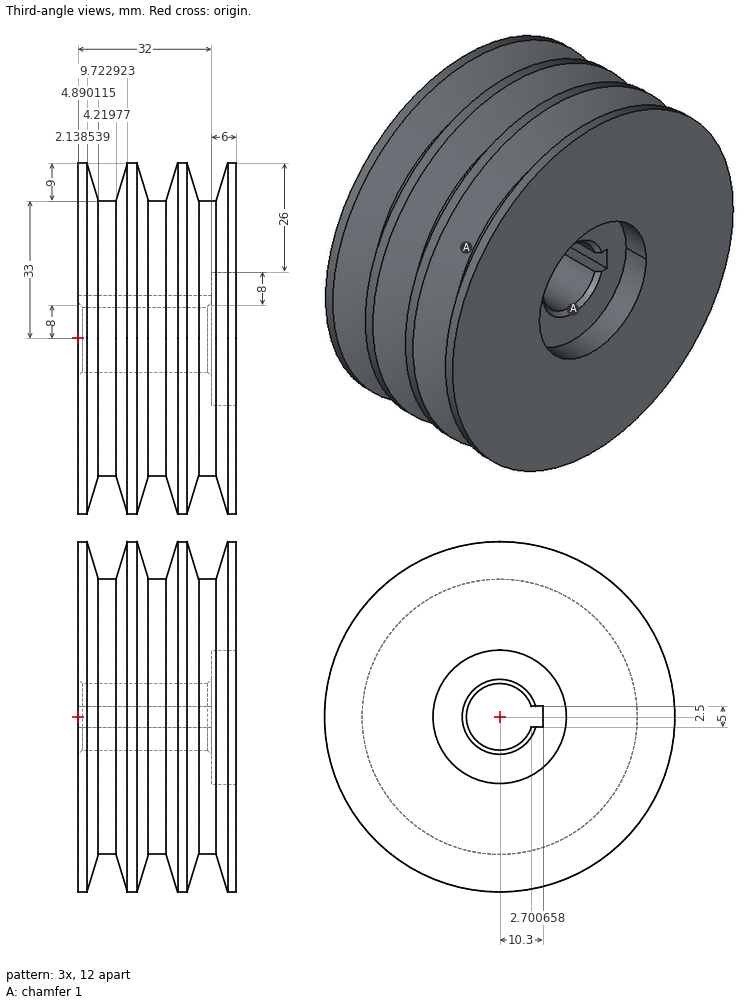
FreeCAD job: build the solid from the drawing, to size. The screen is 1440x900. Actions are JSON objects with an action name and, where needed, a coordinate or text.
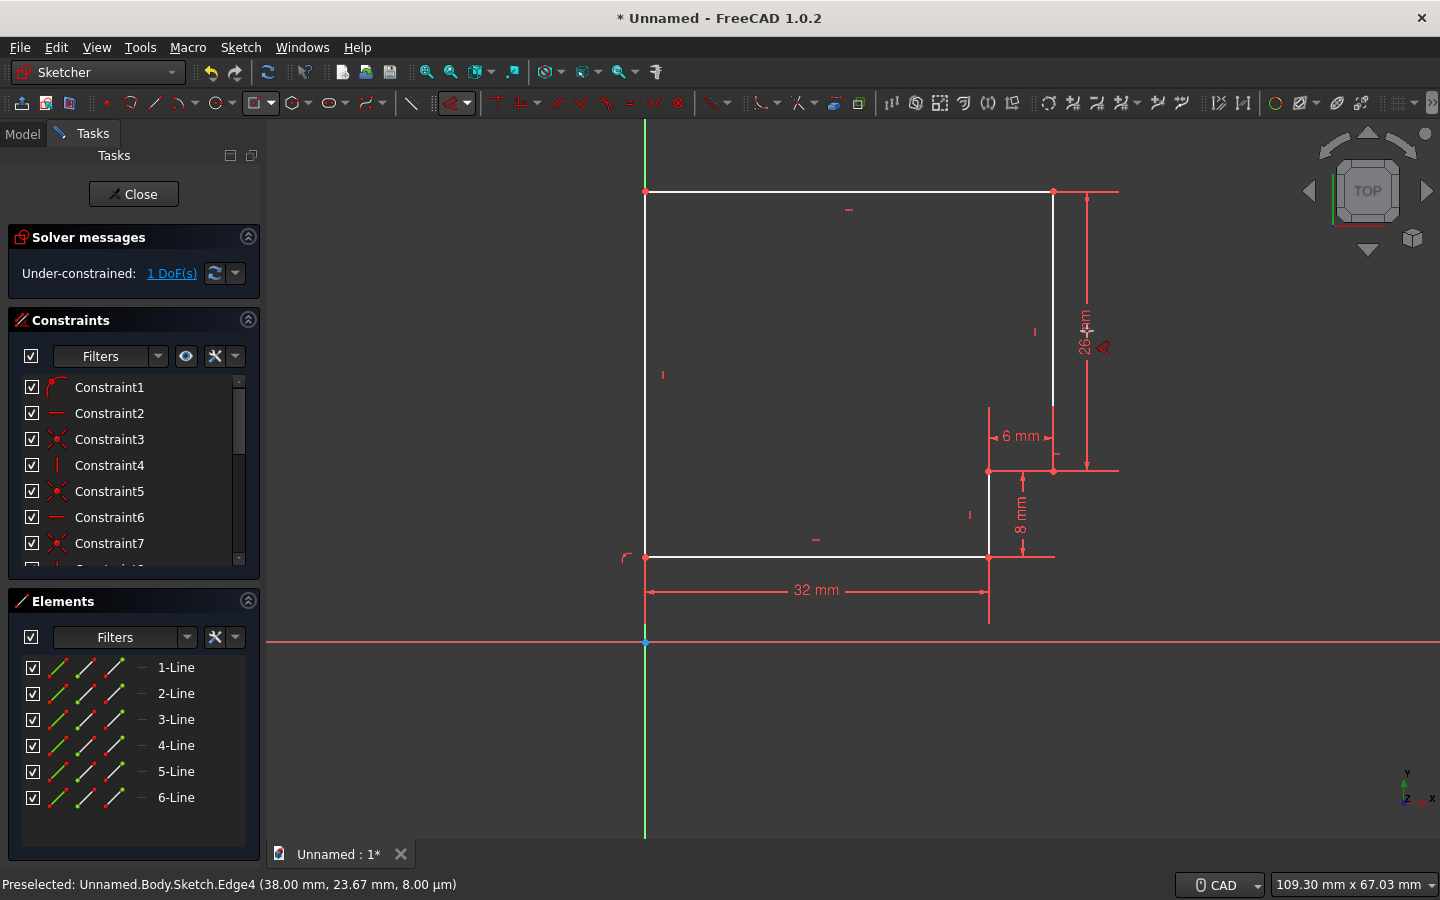
{"action": "left_click", "coordinate": [645, 557]}
{"action": "left_click", "coordinate": [611, 600]}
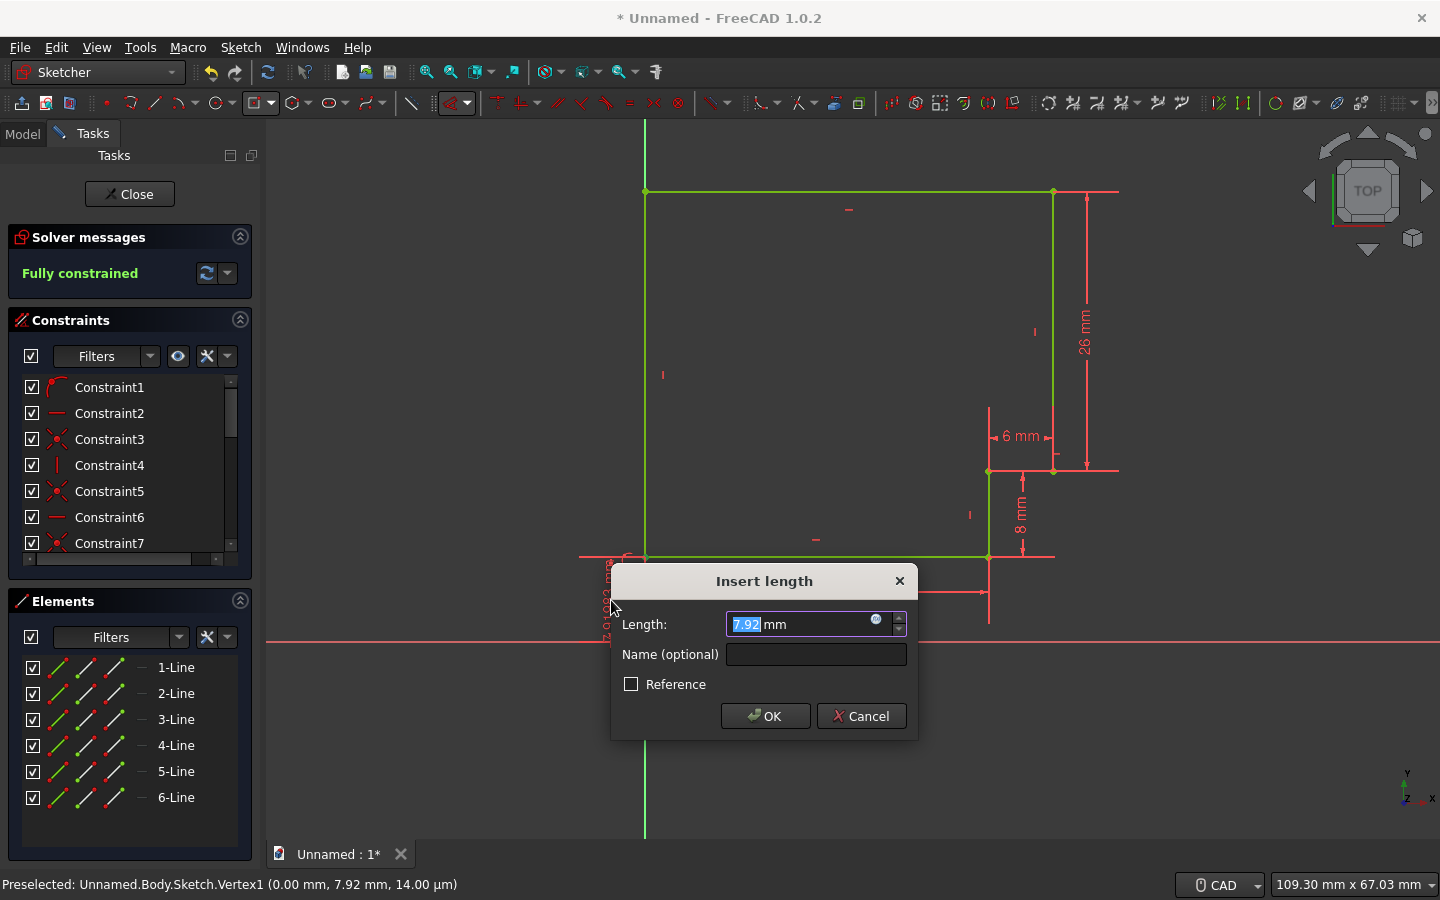
{"action": "type", "text": "8"}
{"action": "key", "text": "Return"}
{"action": "key", "text": "Escape"}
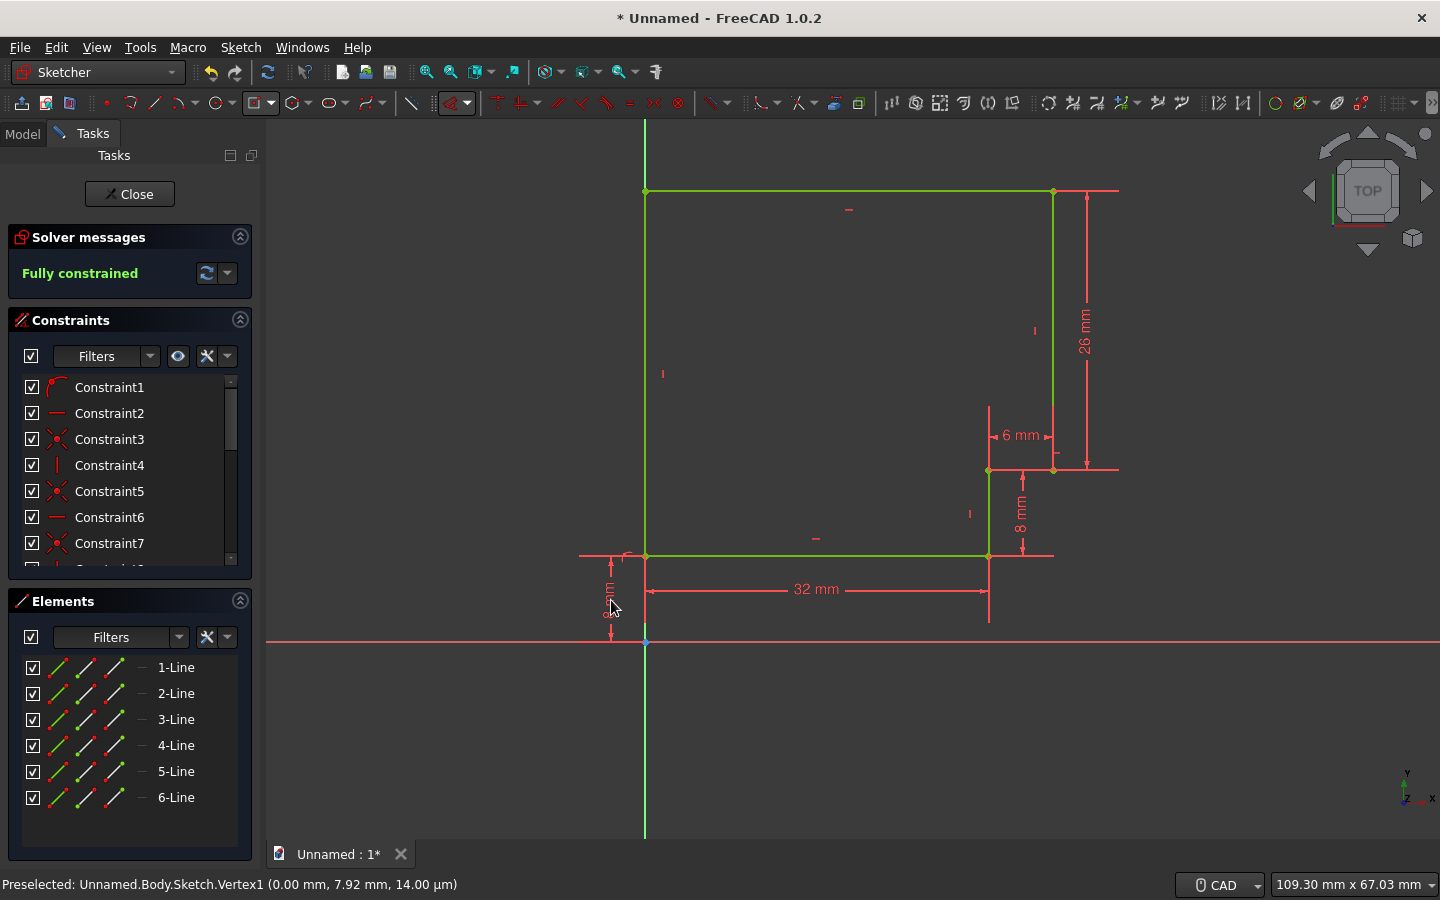
{"action": "left_click", "coordinate": [130, 194]}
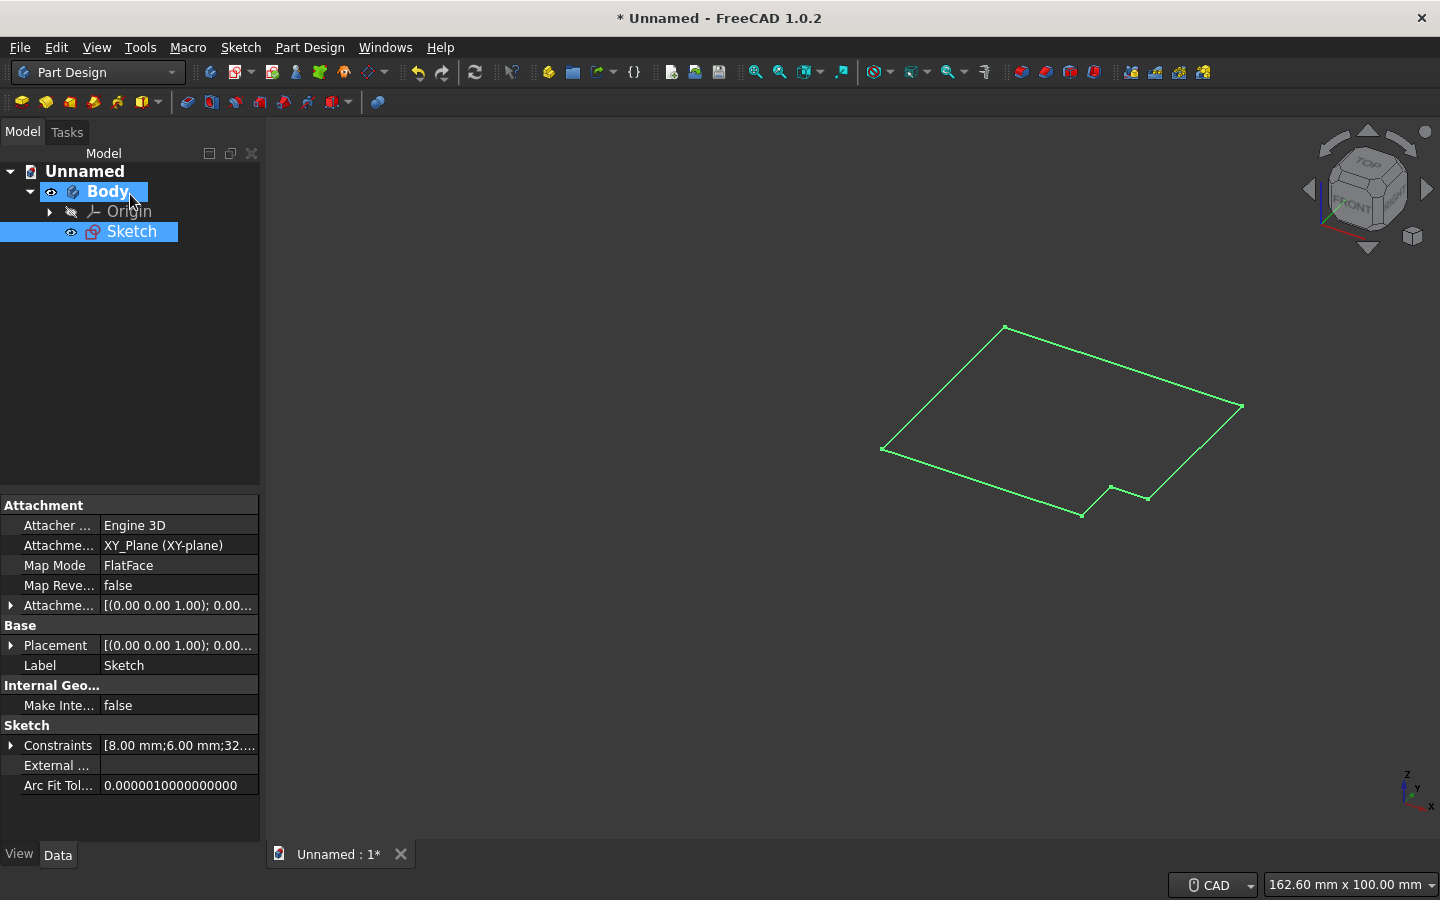
{"action": "left_click", "coordinate": [46, 102]}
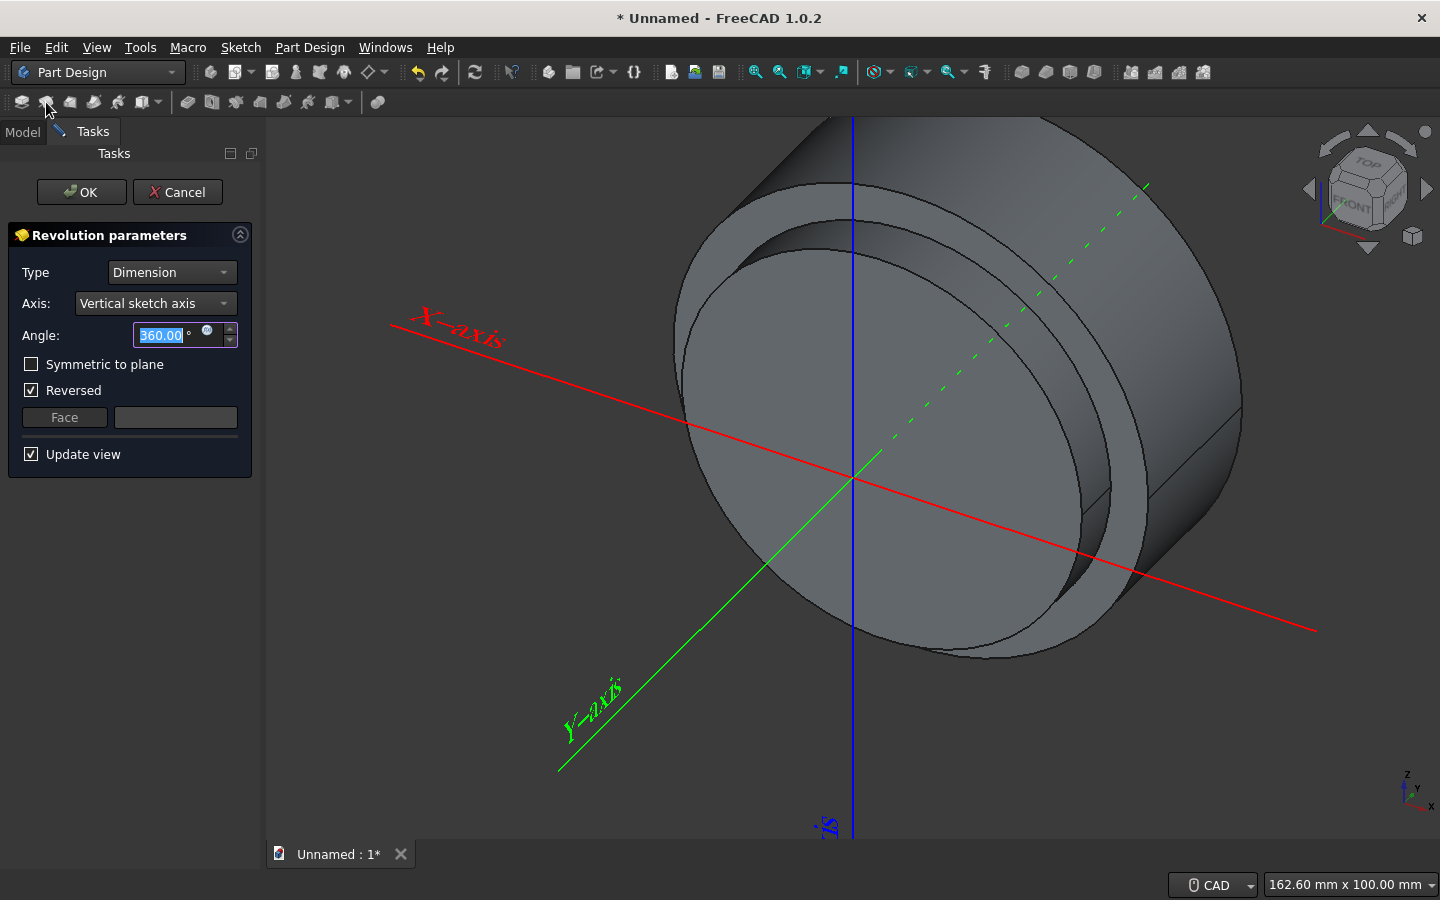
{"action": "left_click", "coordinate": [156, 304]}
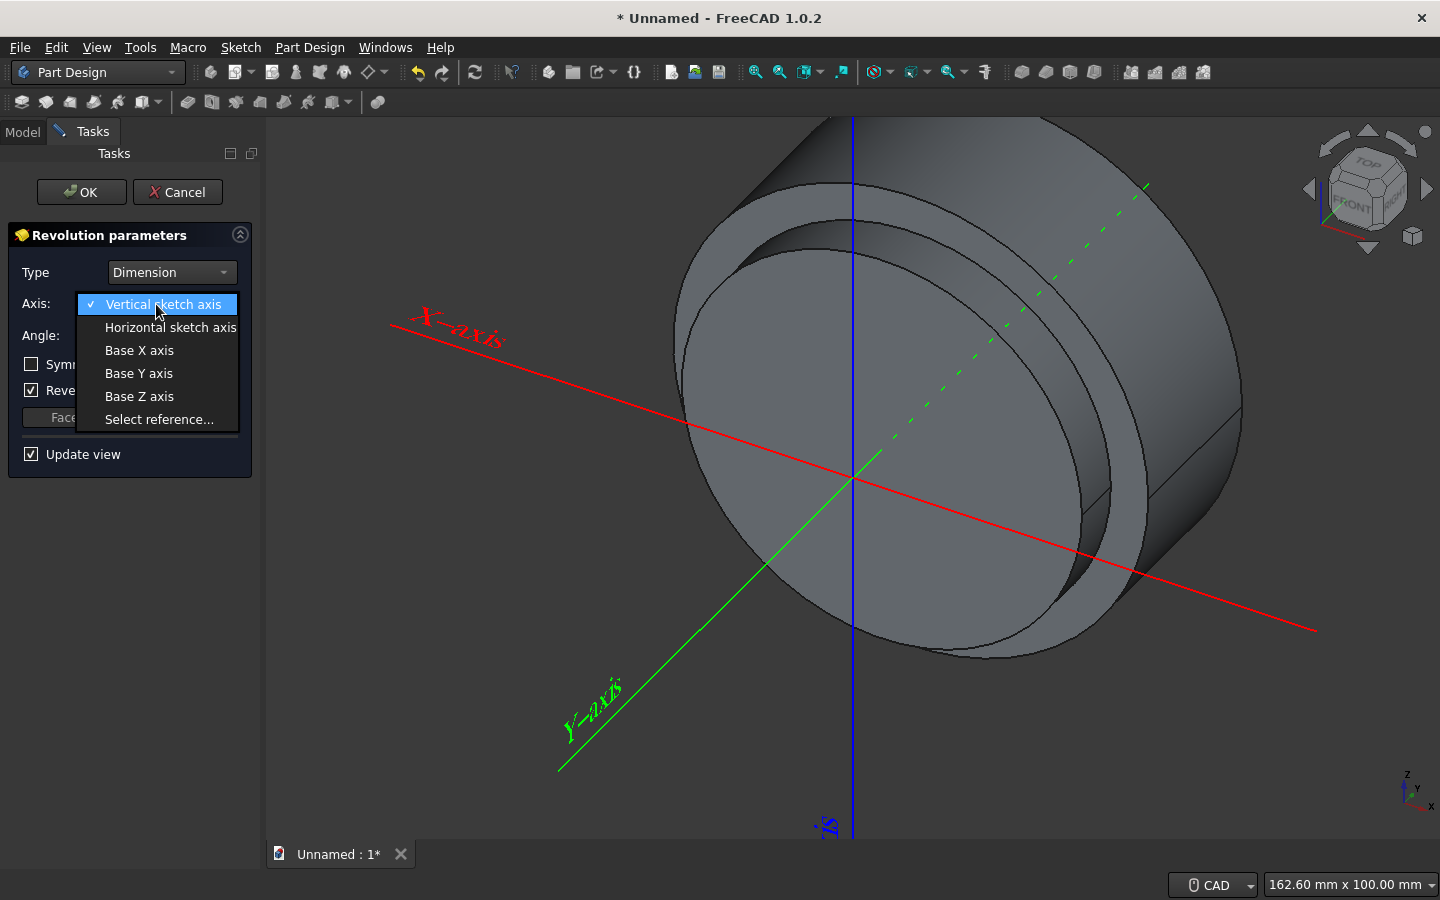
{"action": "left_click", "coordinate": [156, 328]}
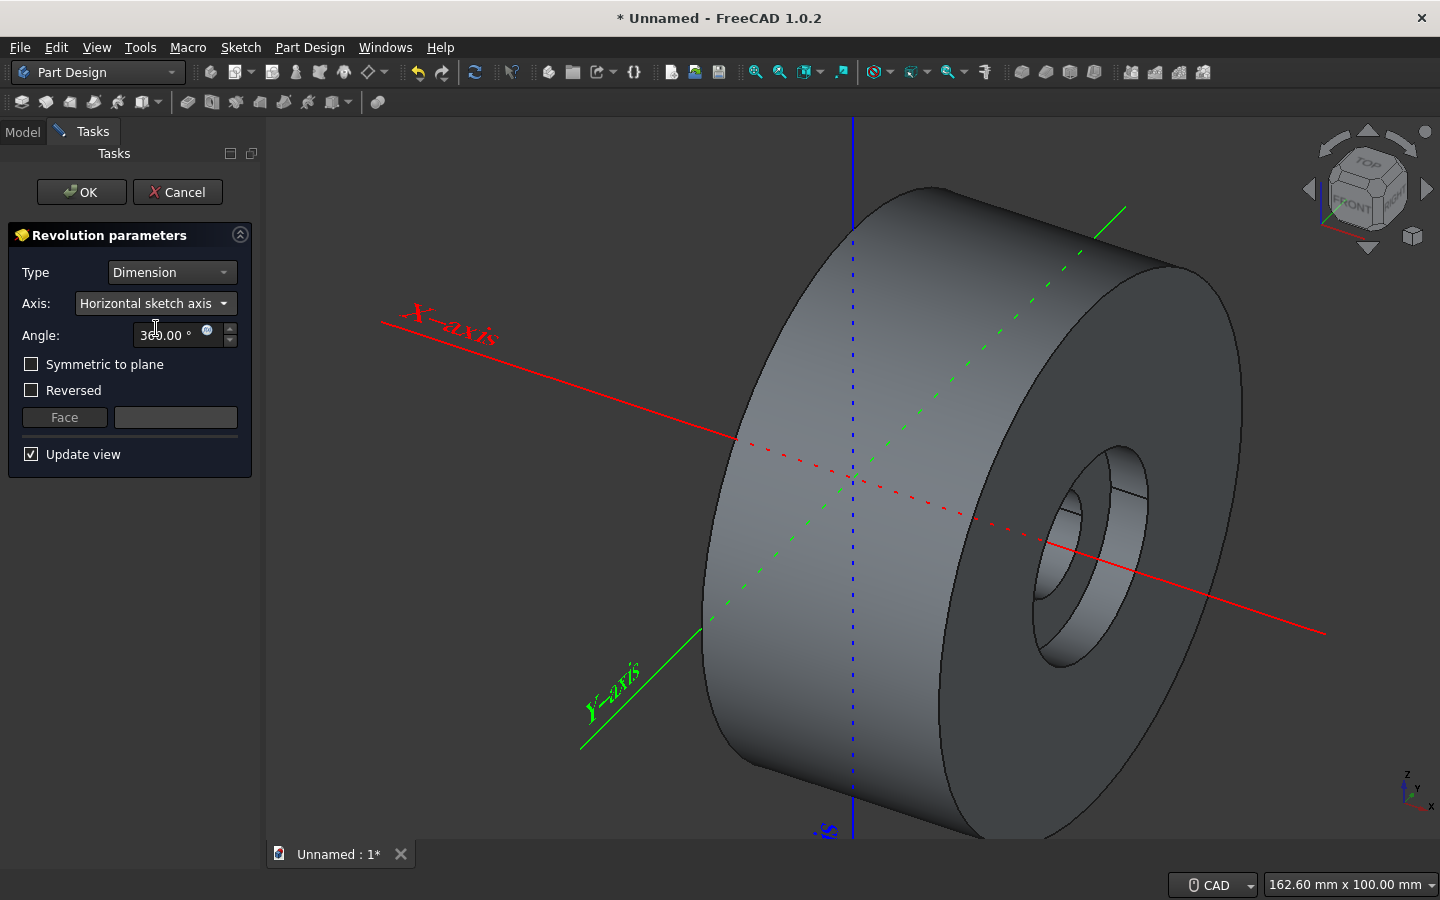
{"action": "left_click", "coordinate": [82, 192]}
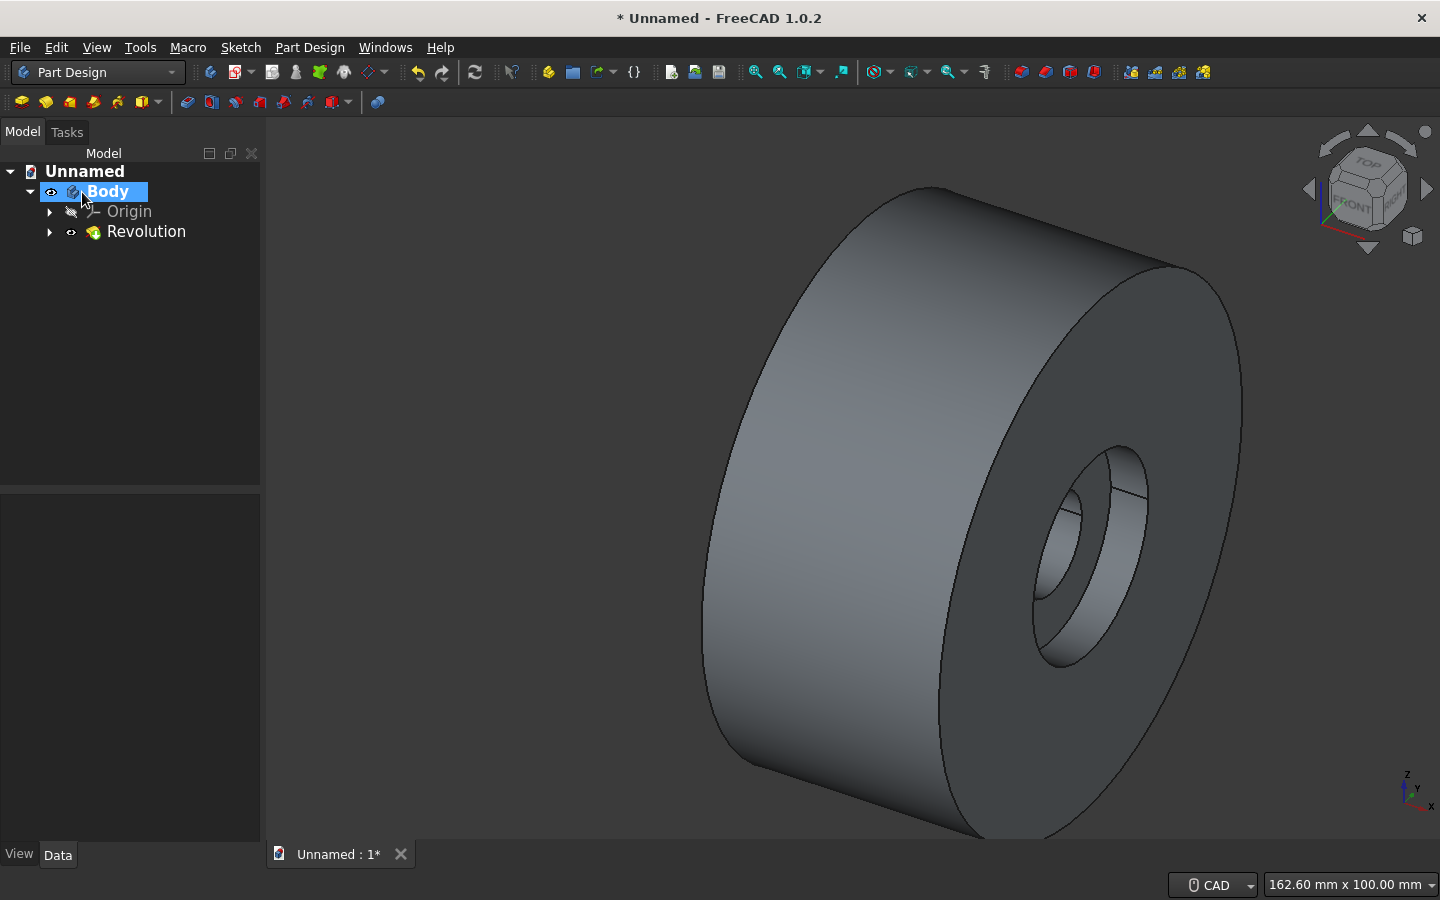
{"action": "key", "text": "v f"}